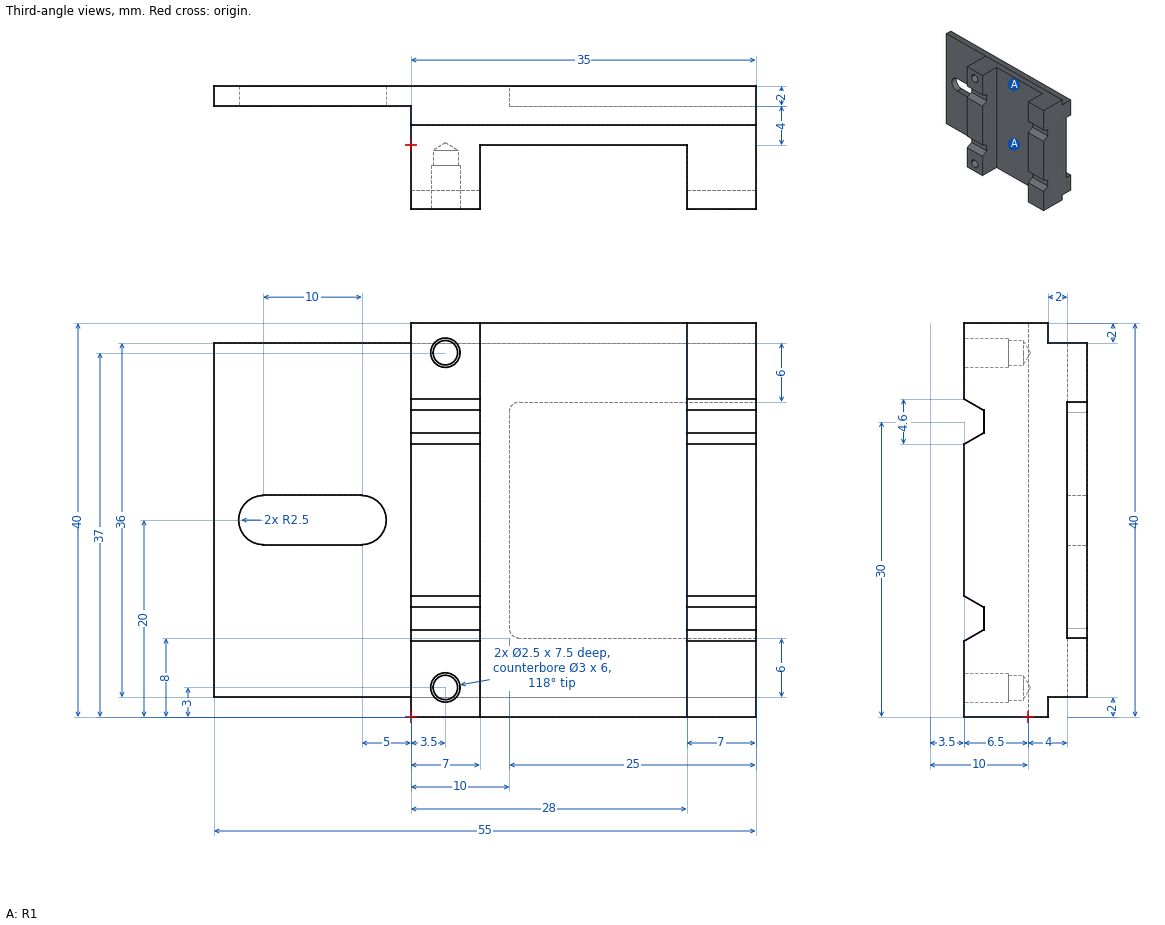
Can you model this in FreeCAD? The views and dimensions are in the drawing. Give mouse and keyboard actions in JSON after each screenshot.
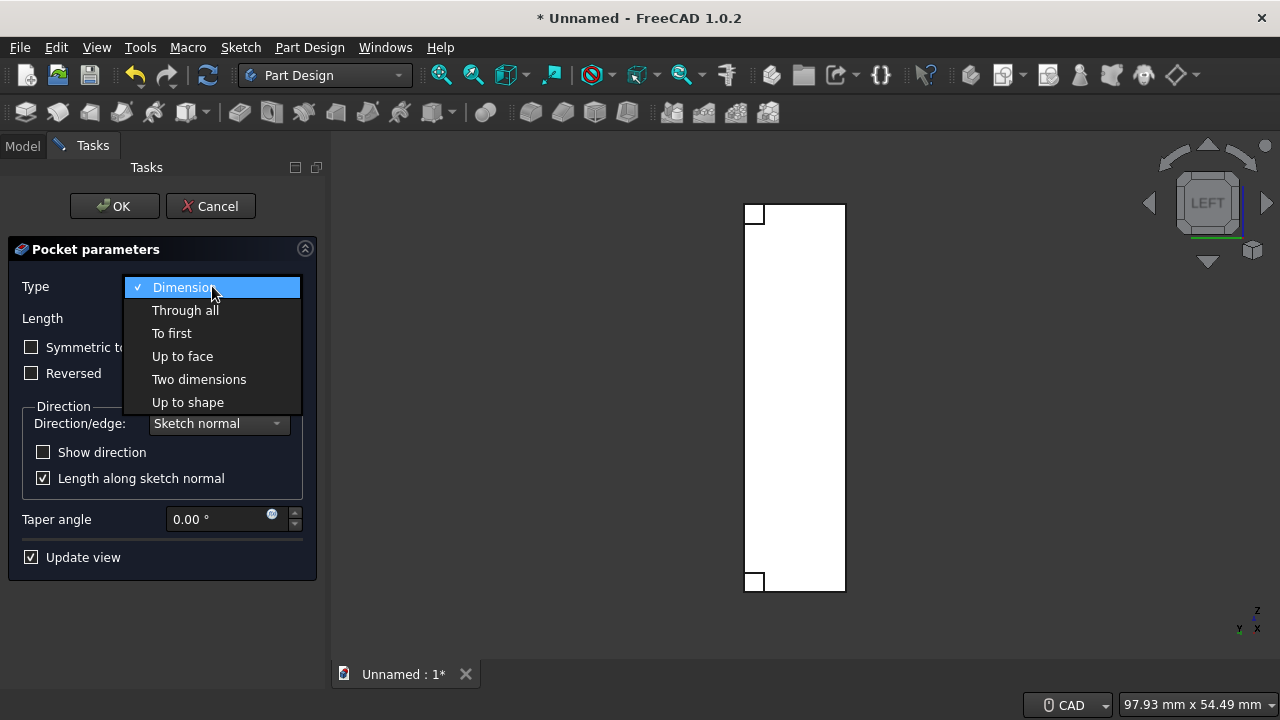
{"action": "left_click", "coordinate": [212, 310]}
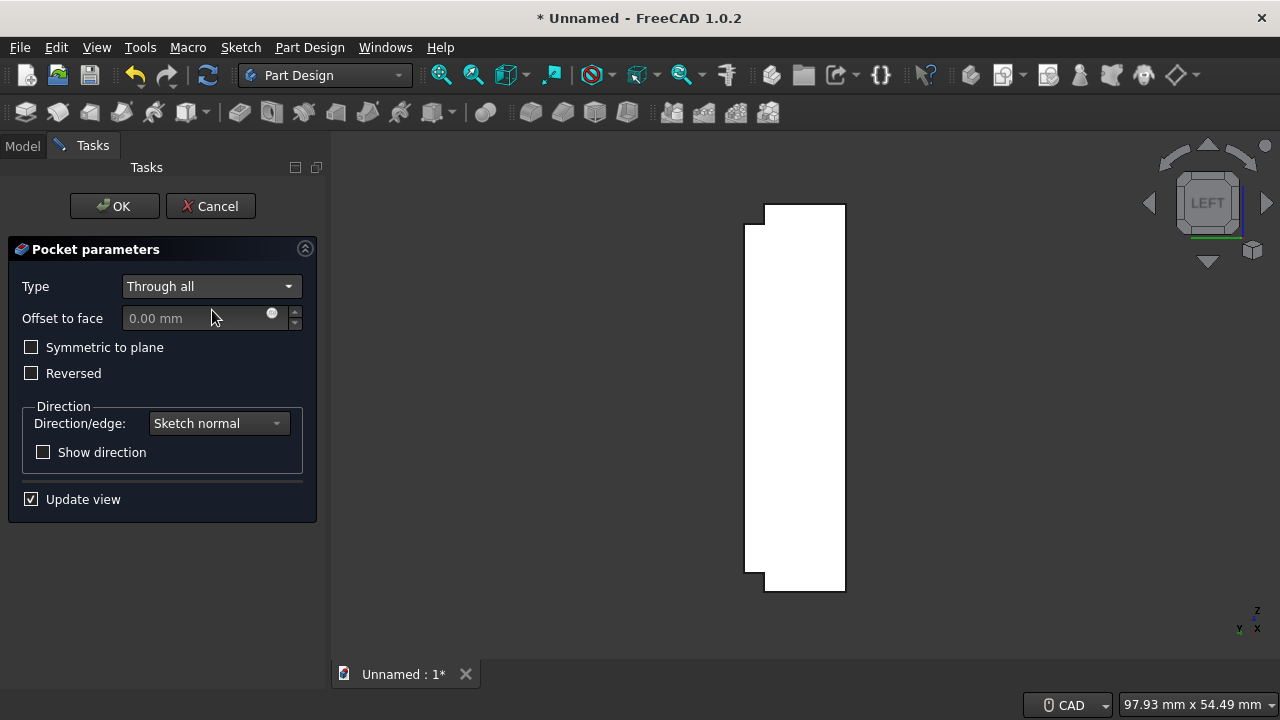
{"action": "left_click", "coordinate": [115, 206]}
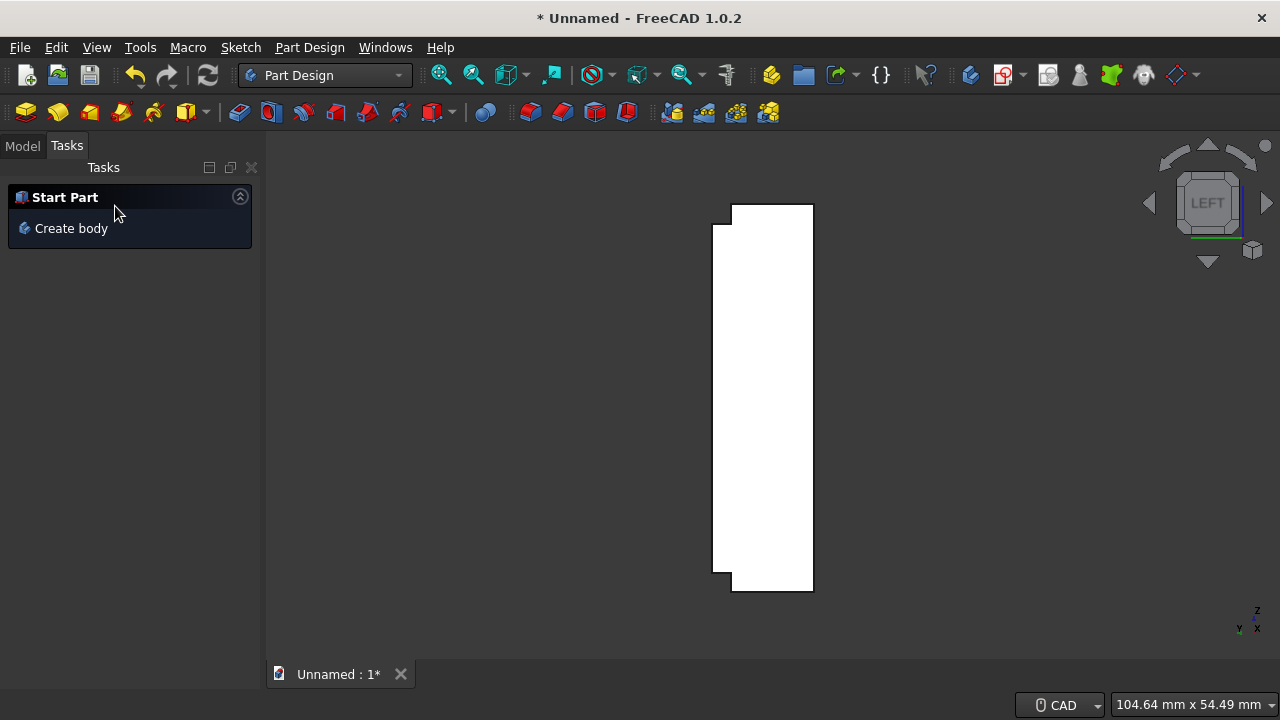
{"action": "key", "text": "4"}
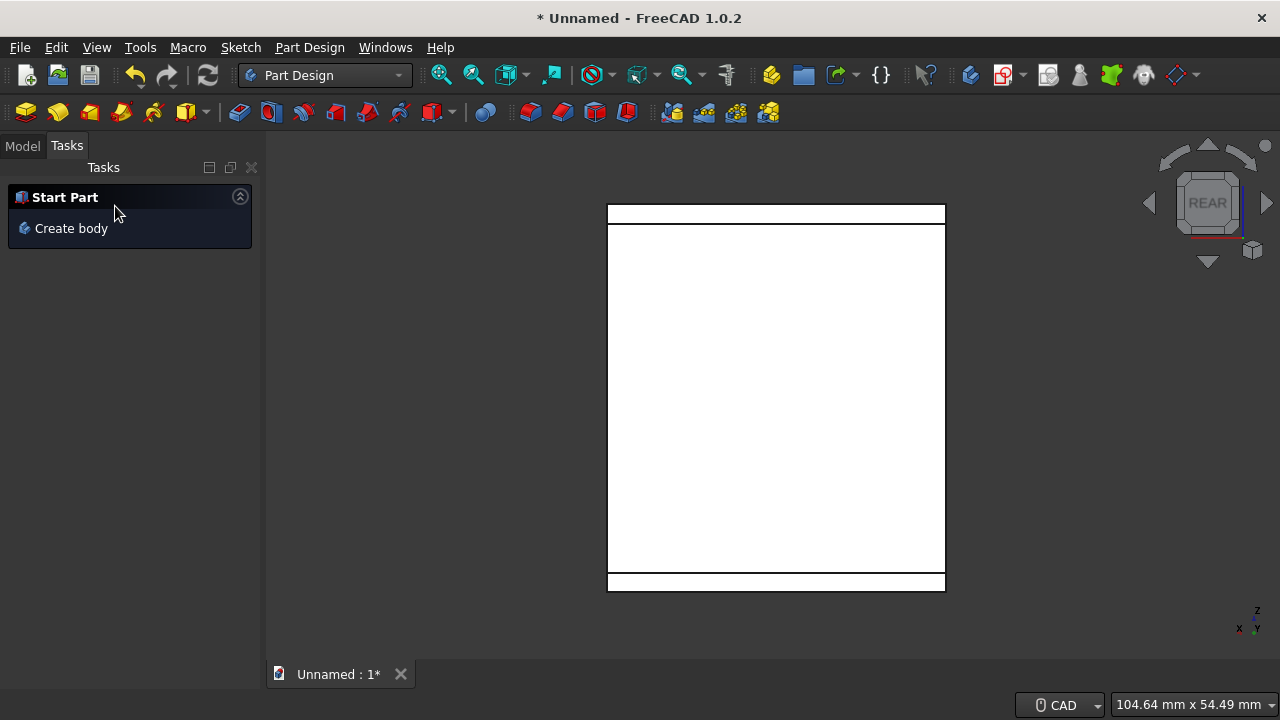
{"action": "left_click", "coordinate": [776, 397]}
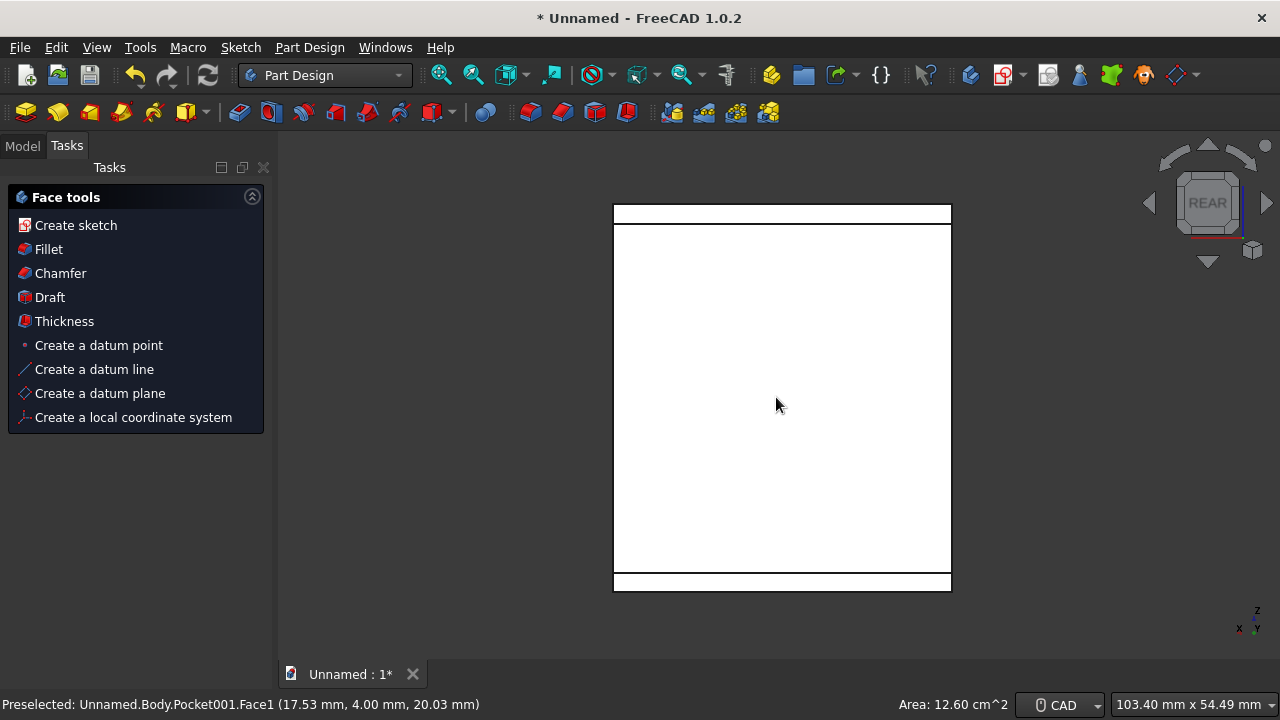
{"action": "left_click", "coordinate": [1004, 76]}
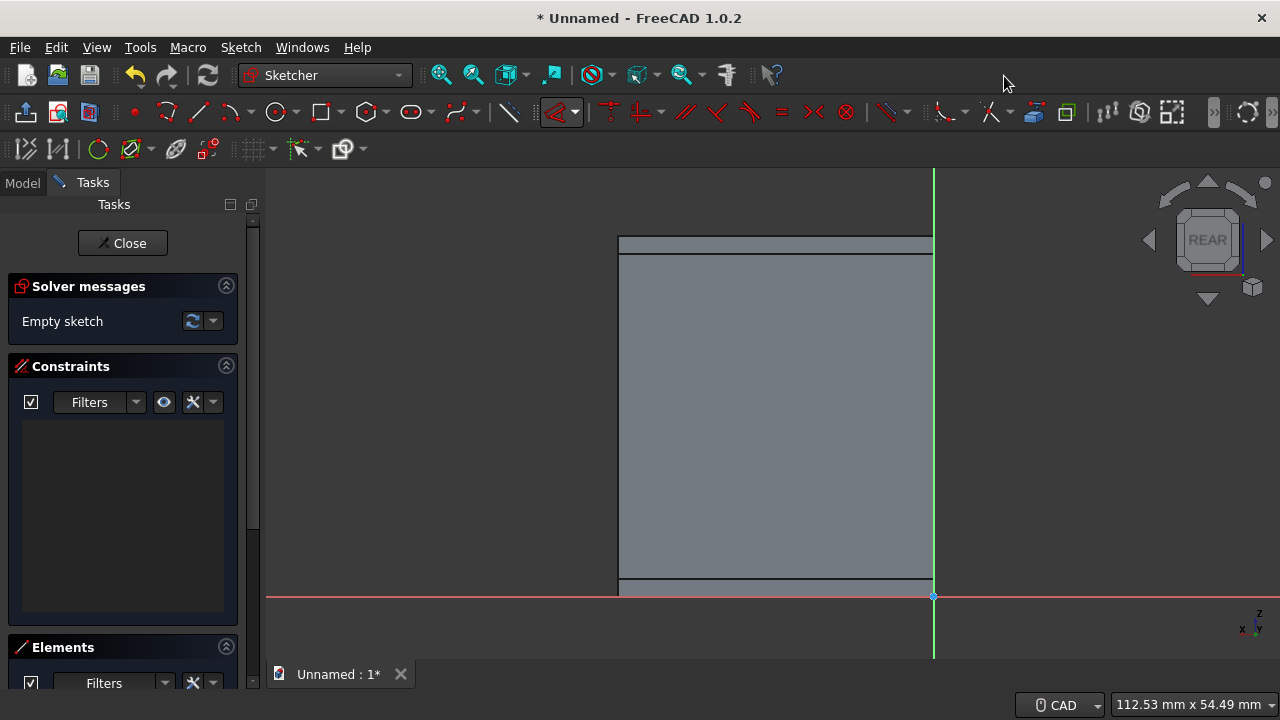
{"action": "scroll", "coordinate": [294, 359], "scroll_direction": "down", "scroll_amount": 1}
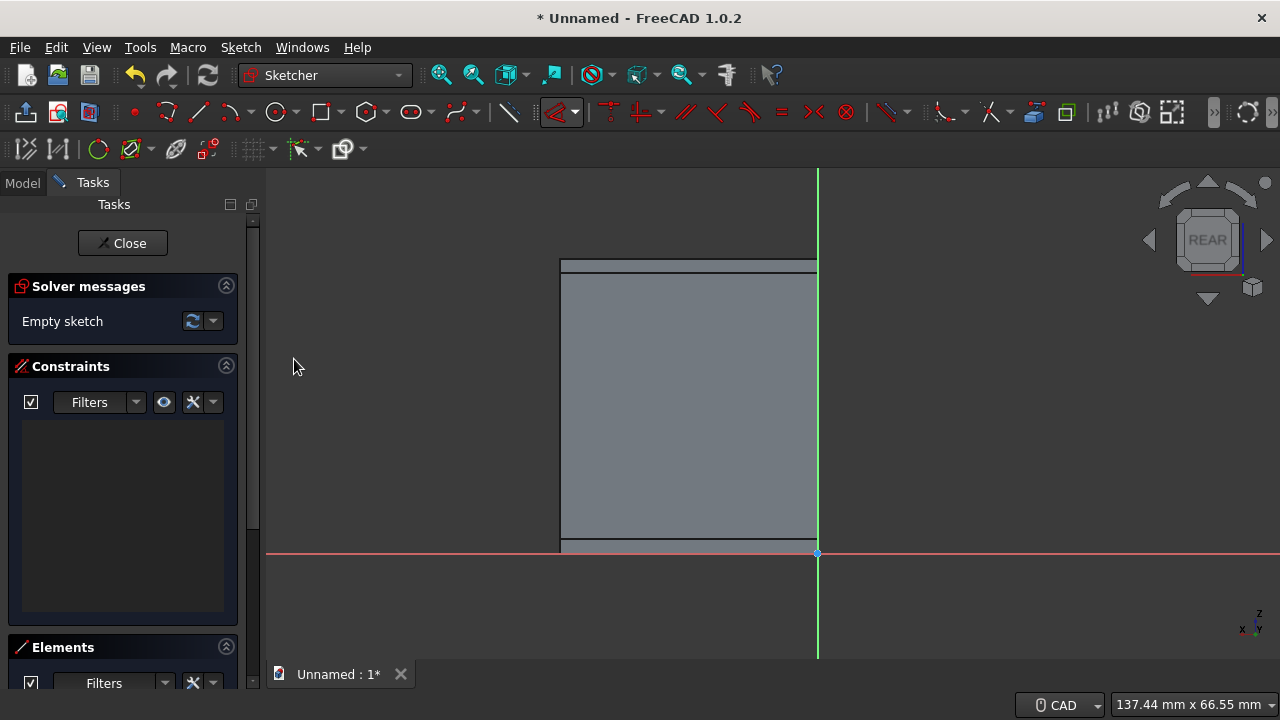
{"action": "left_click", "coordinate": [168, 112]}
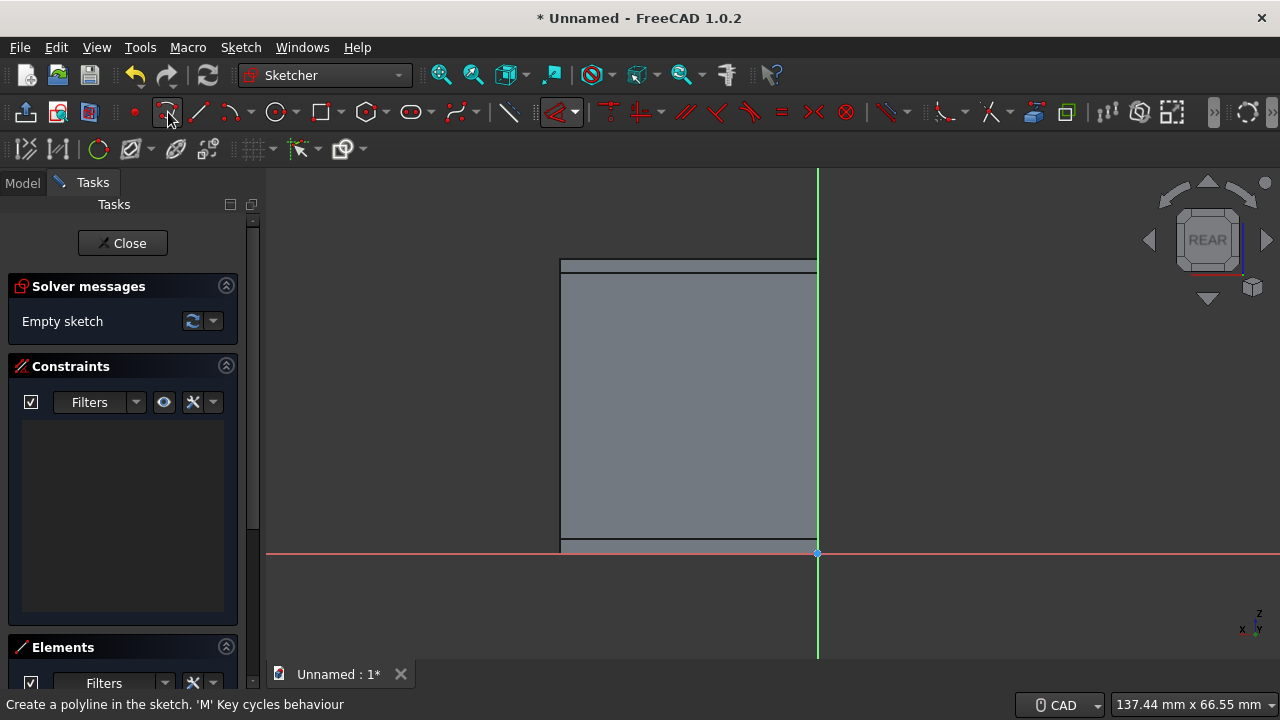
{"action": "left_click", "coordinate": [744, 495]}
{"action": "left_click", "coordinate": [560, 495]}
{"action": "left_click", "coordinate": [560, 539]}
{"action": "left_click", "coordinate": [965, 539]}
{"action": "left_click", "coordinate": [965, 273]}
{"action": "left_click", "coordinate": [560, 273]}
{"action": "left_click", "coordinate": [560, 318]}
{"action": "left_click", "coordinate": [744, 318]}
{"action": "left_click", "coordinate": [744, 496]}
{"action": "key", "text": "Escape"}
{"action": "key", "text": "Escape"}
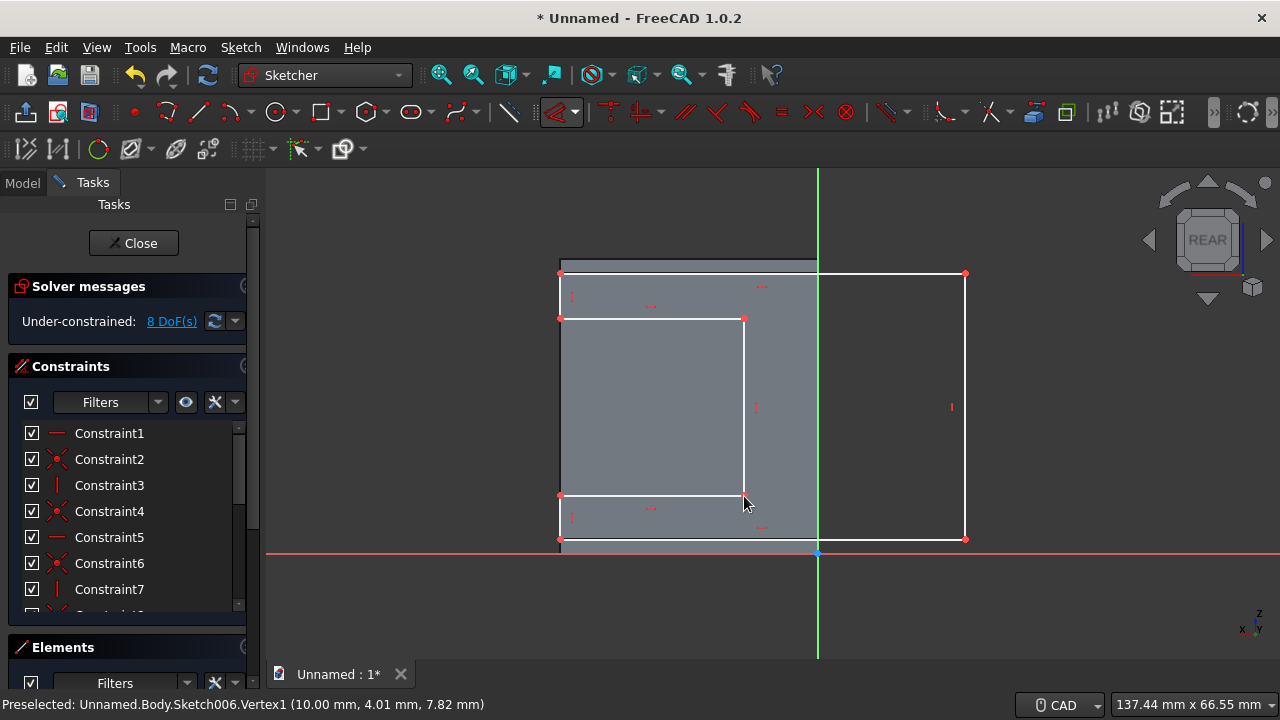
{"action": "left_click", "coordinate": [560, 509]}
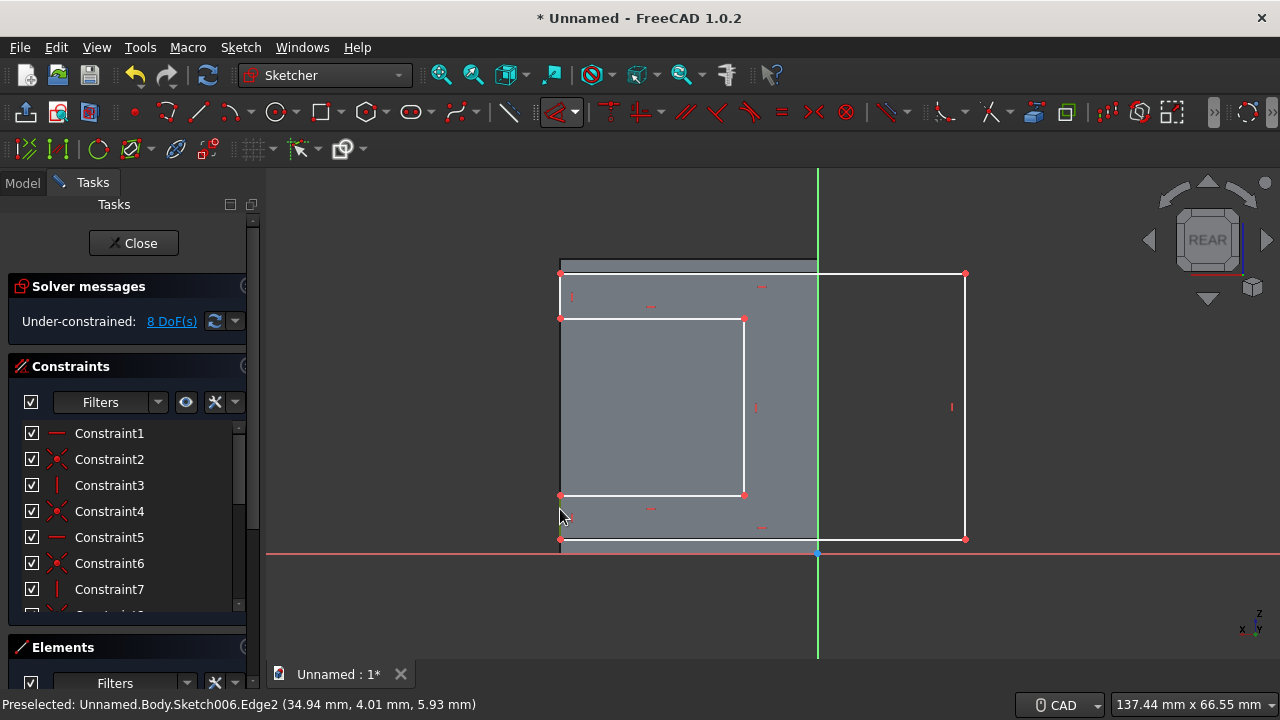
{"action": "key", "text": "i"}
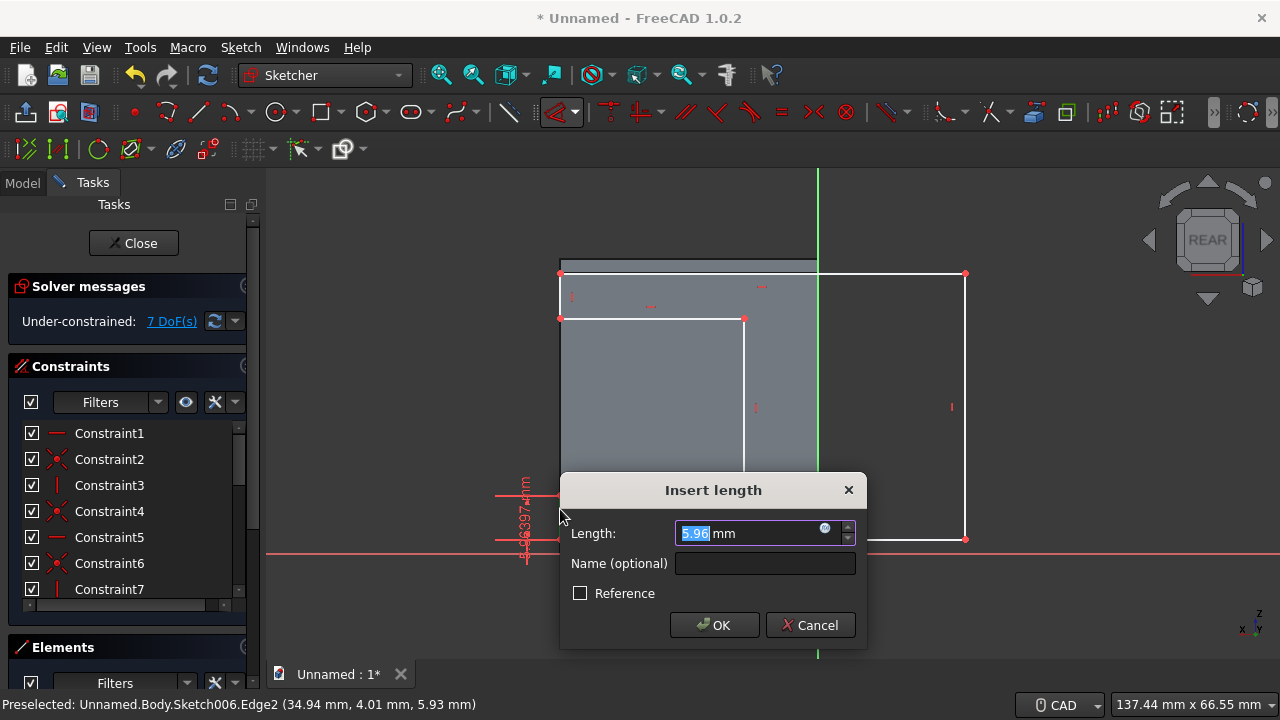
{"action": "type", "text": "6"}
{"action": "key", "text": "Return"}